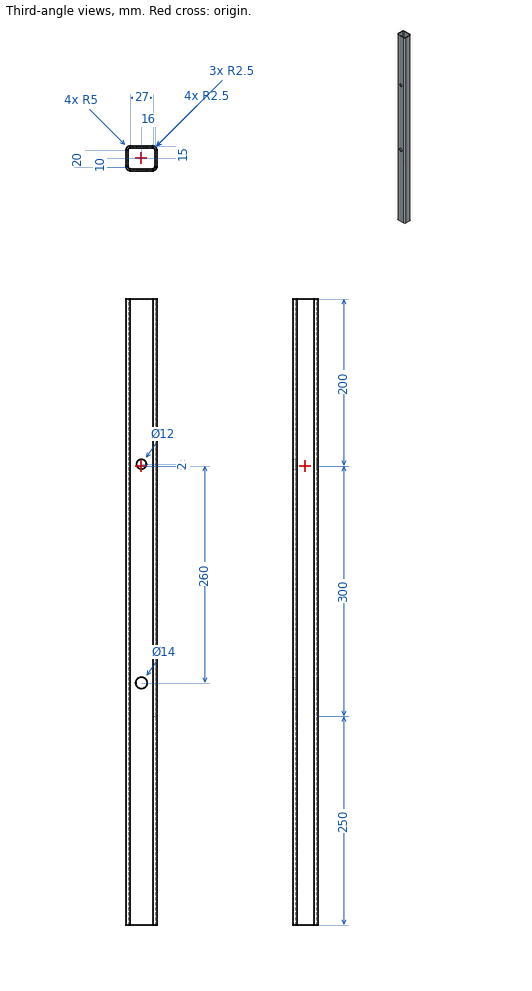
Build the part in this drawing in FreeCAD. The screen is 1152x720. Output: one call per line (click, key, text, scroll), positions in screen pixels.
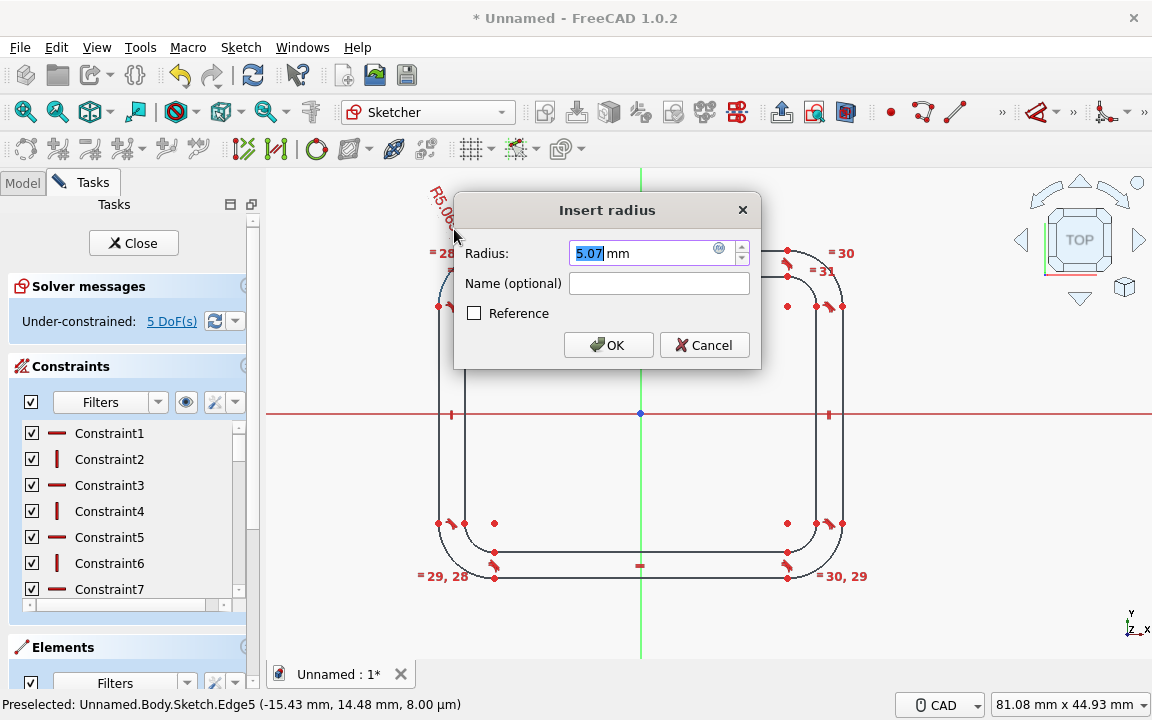
text(5)
key(Return)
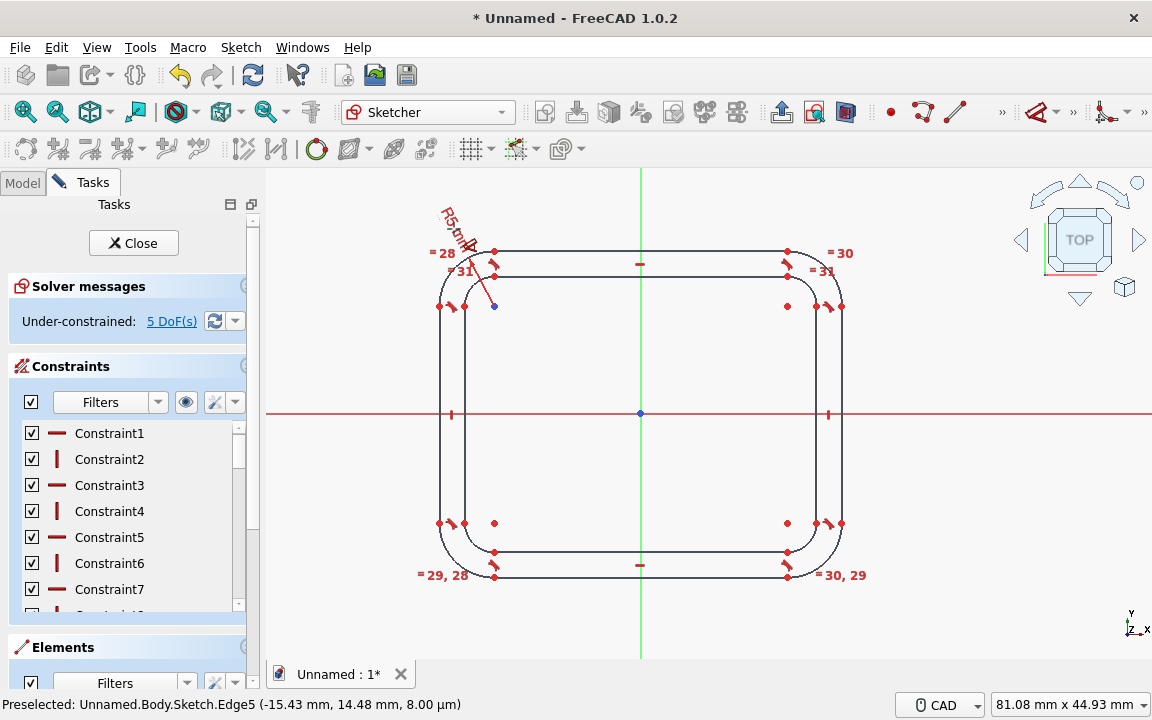
scroll(813, 293, up, 2)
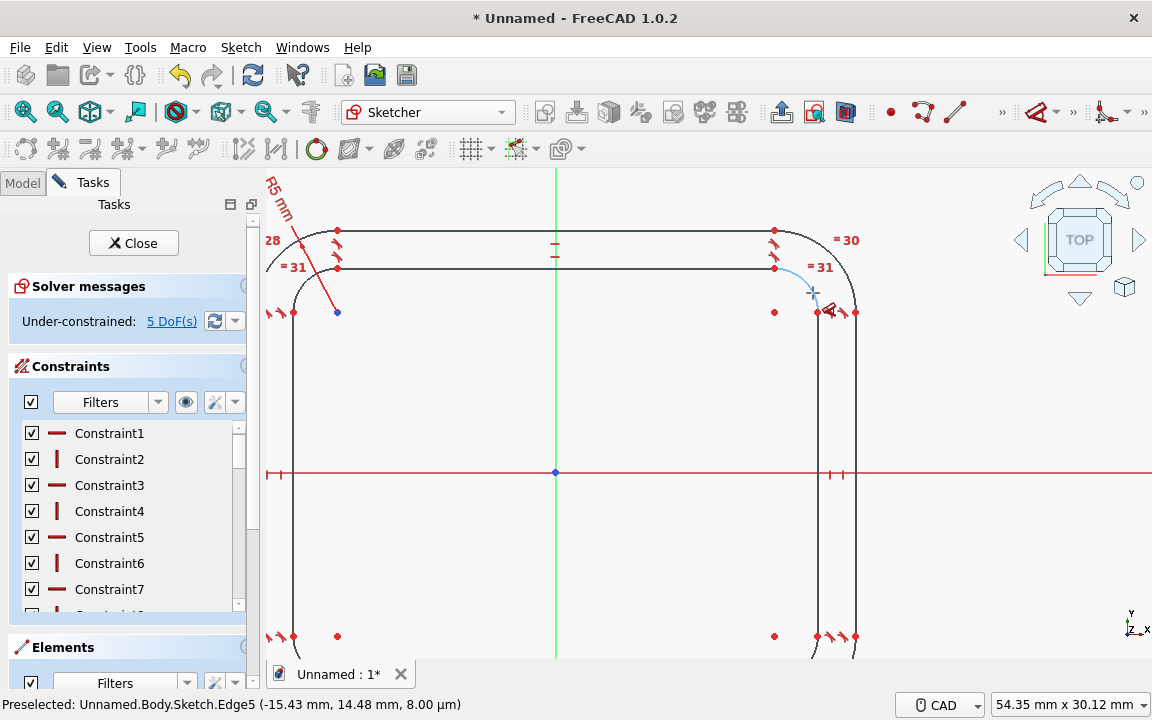
click(813, 293)
click(839, 351)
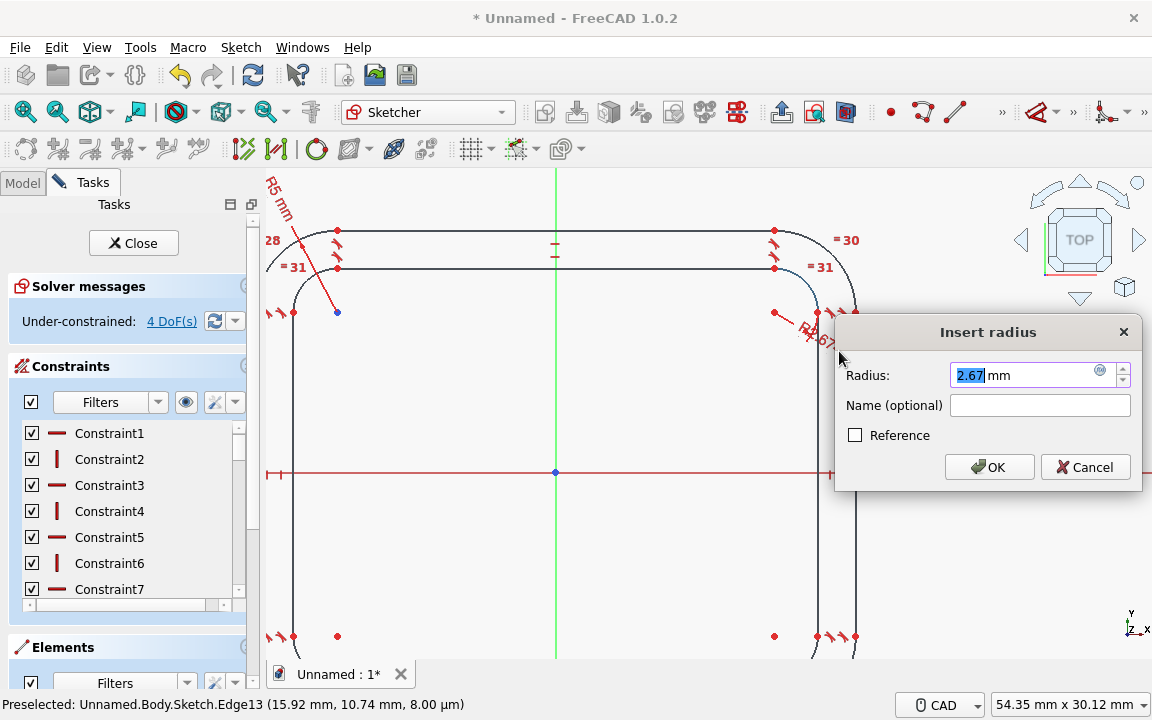
text(2.5)
key(Return)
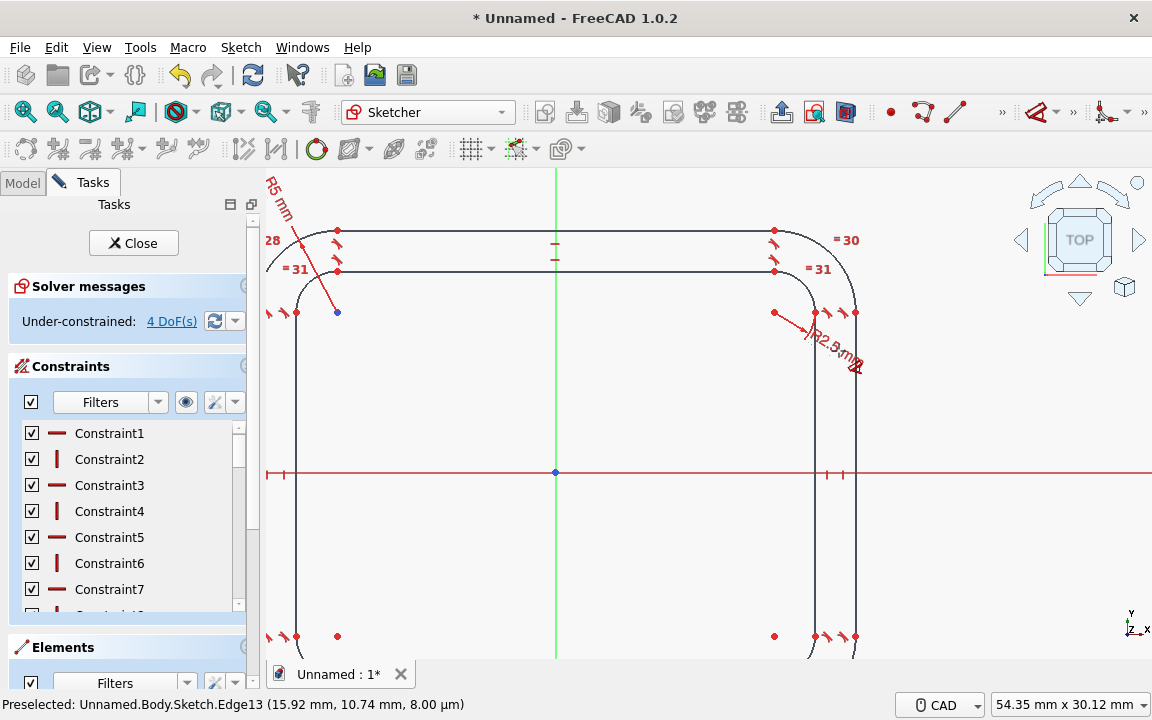
click(643, 231)
click(455, 197)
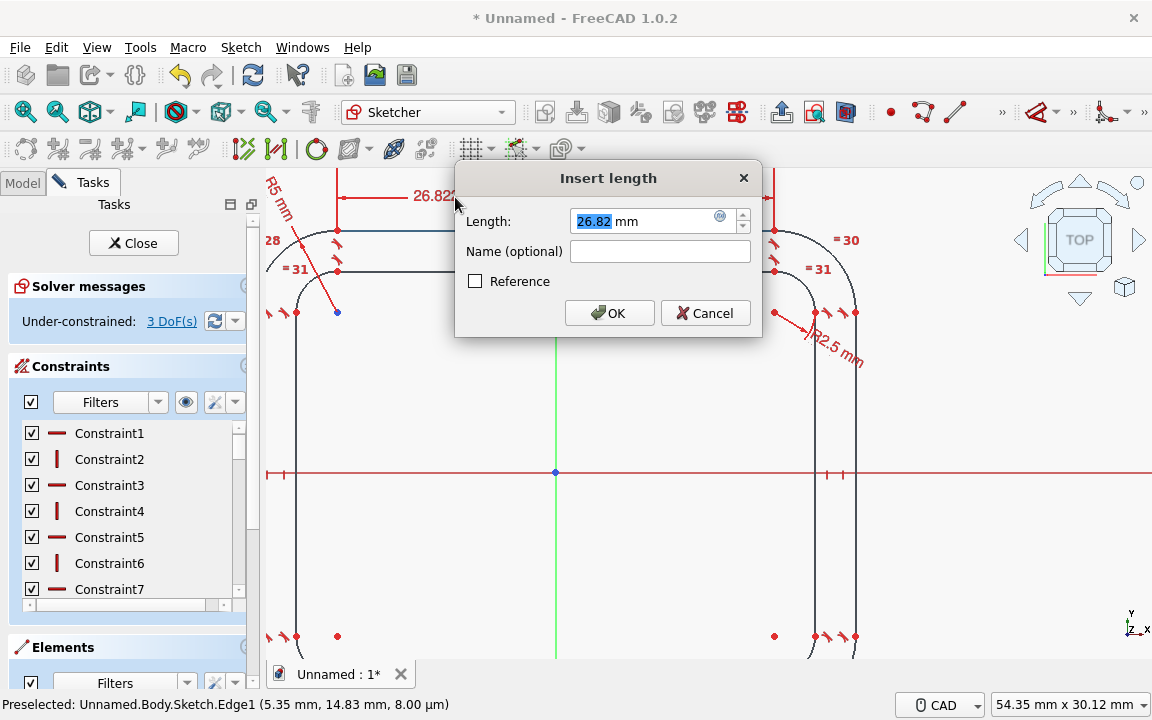
text(27)
key(Return)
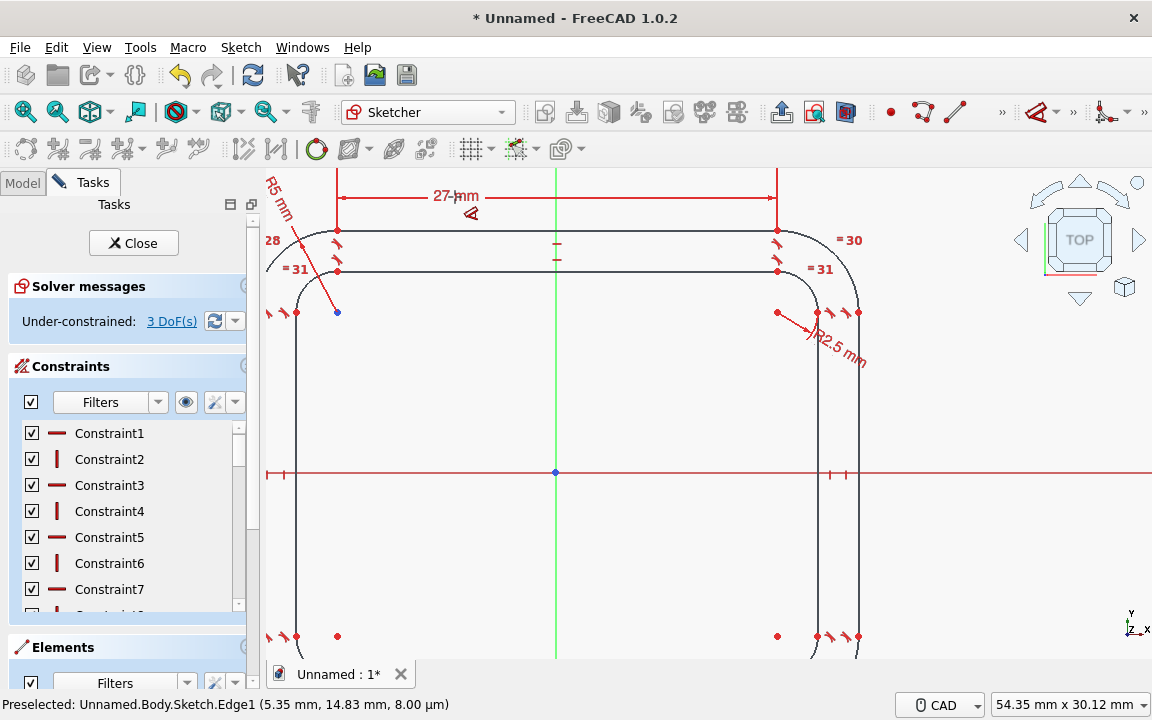
scroll(813, 293, down, 2)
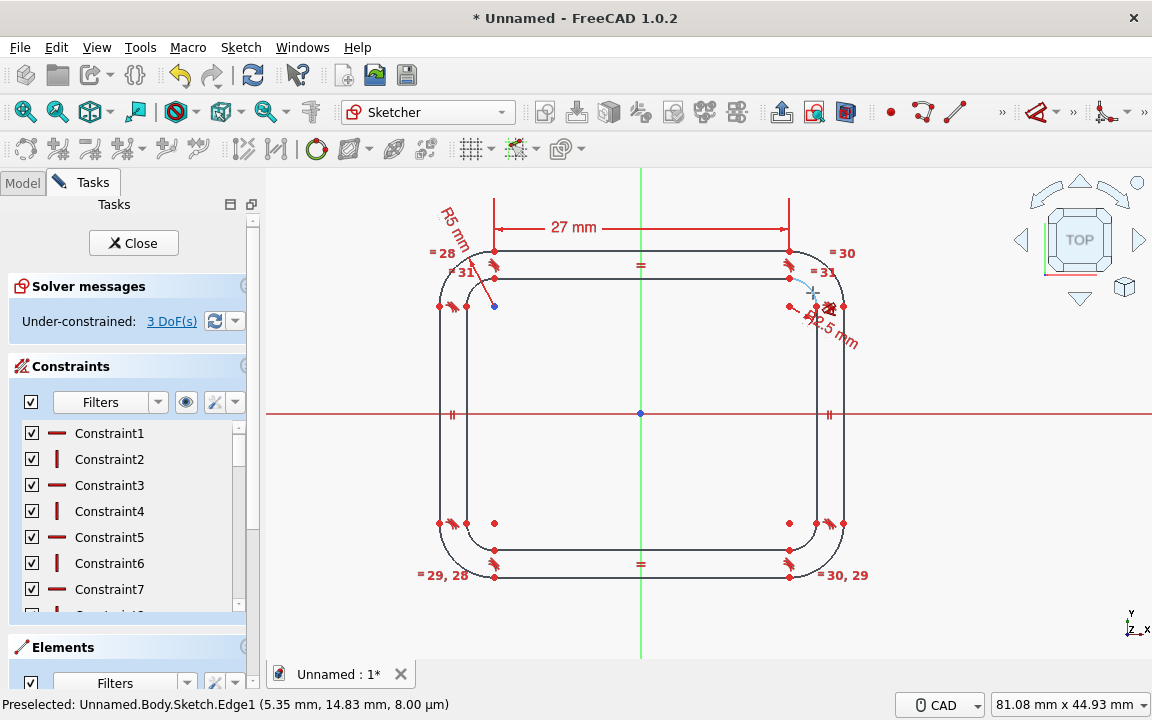
click(440, 371)
click(406, 365)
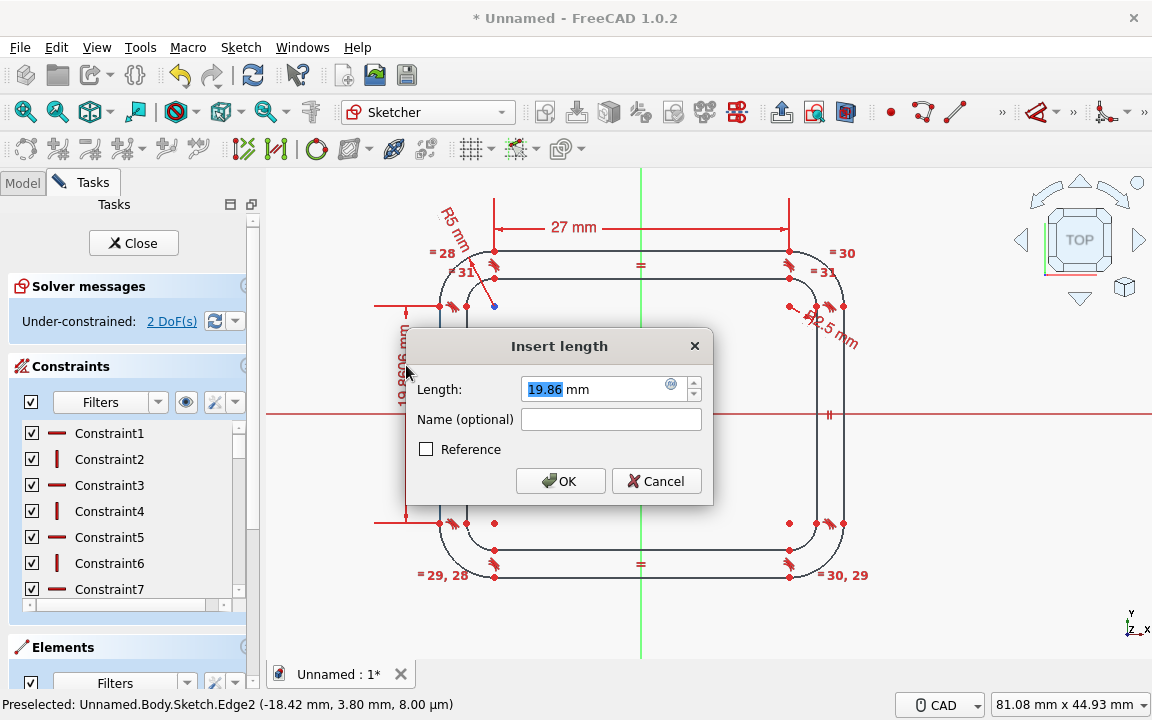
text(20)
key(Return)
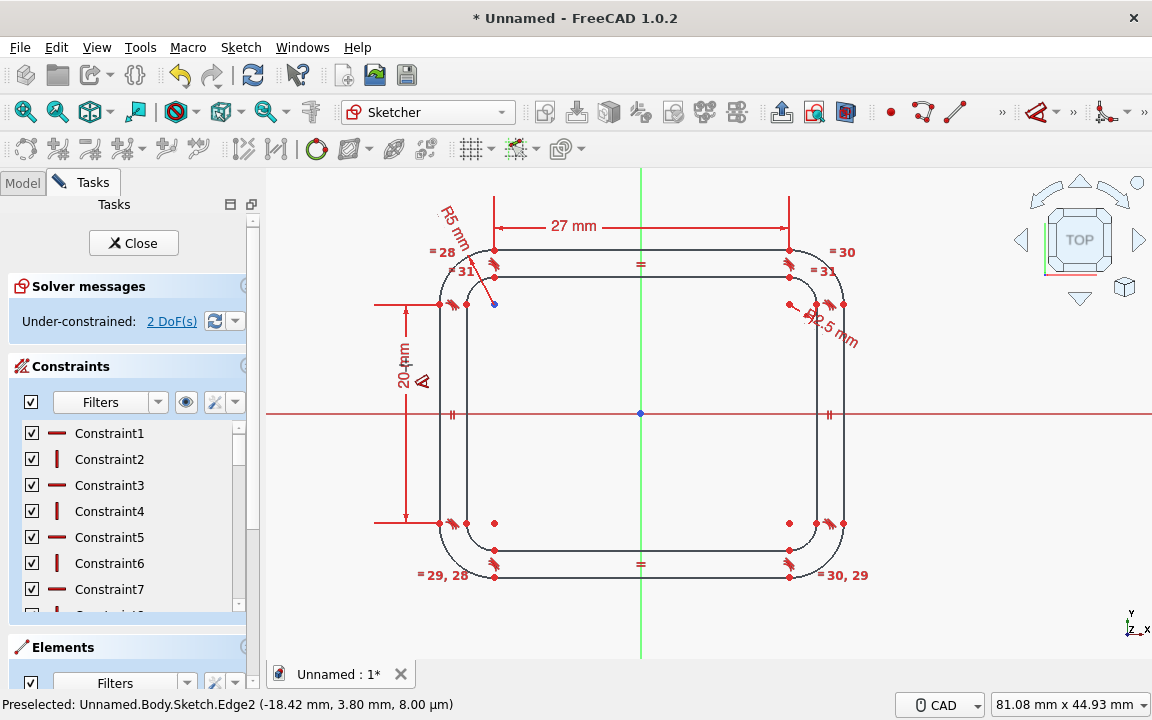
click(789, 250)
click(607, 332)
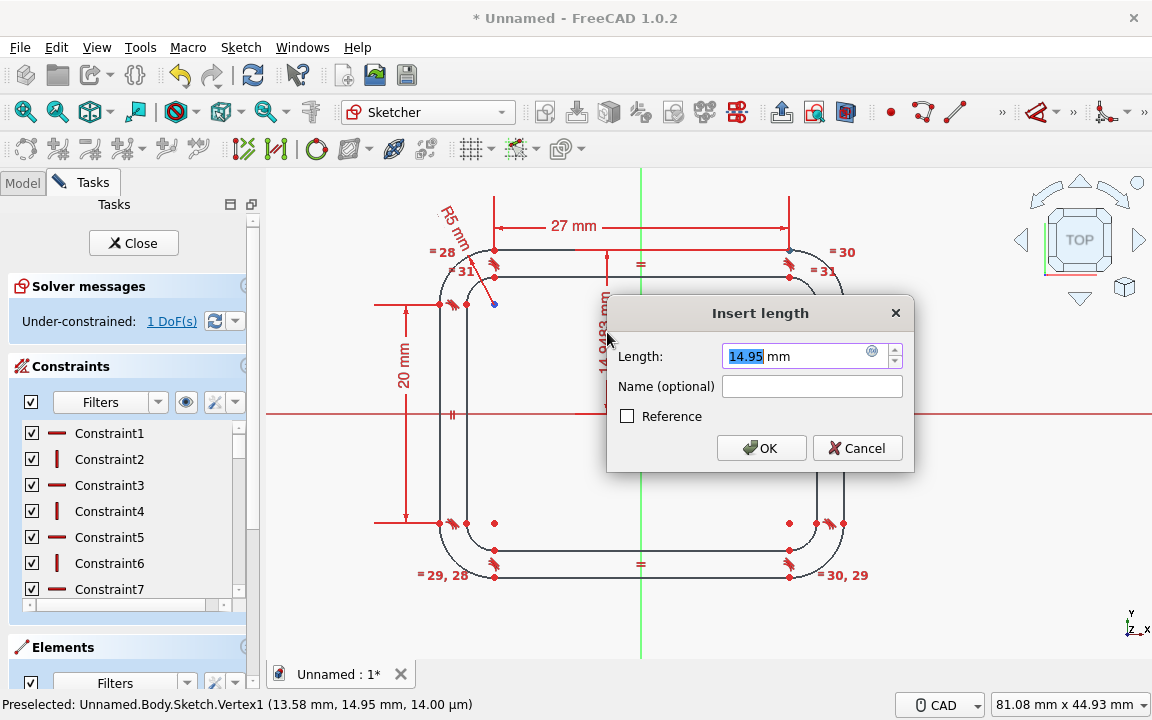
text(15)
key(Return)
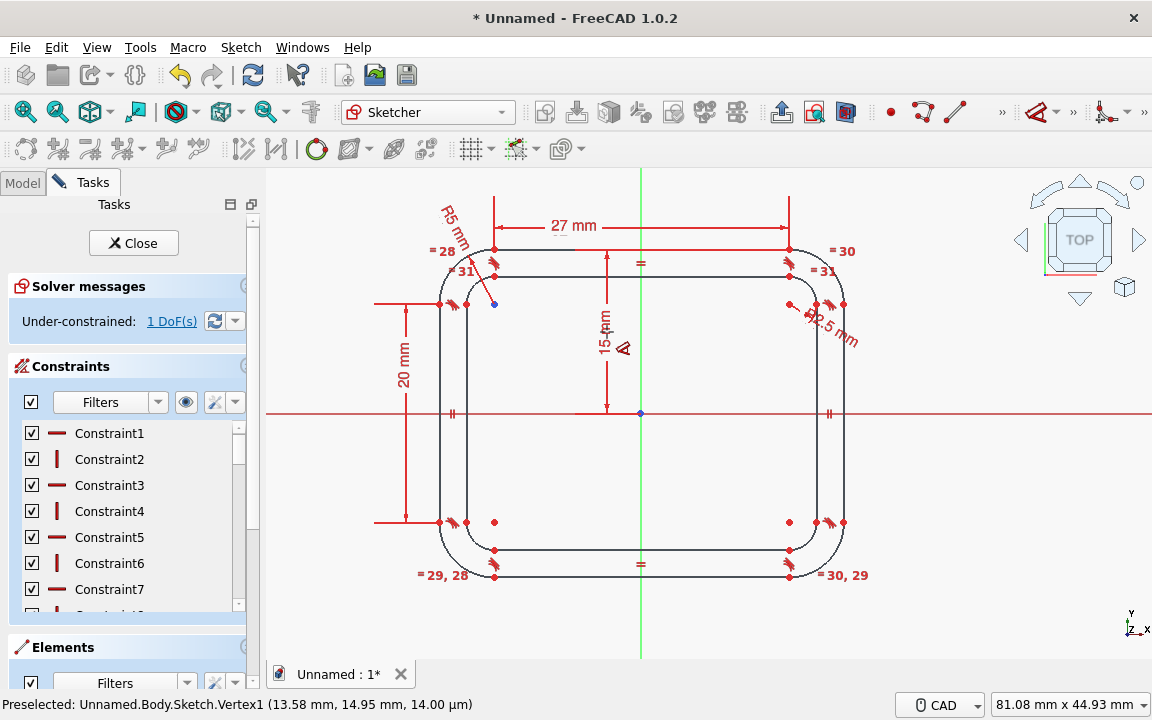
click(817, 304)
click(729, 447)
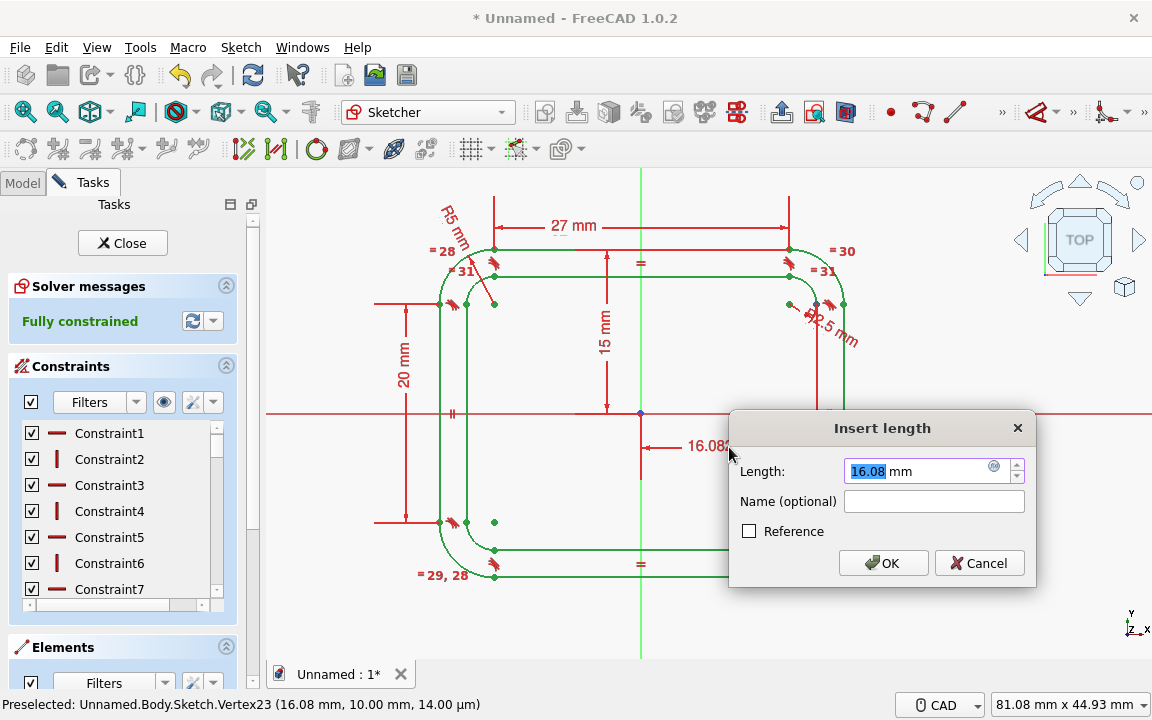
text(16)
key(Return)
key(Escape)